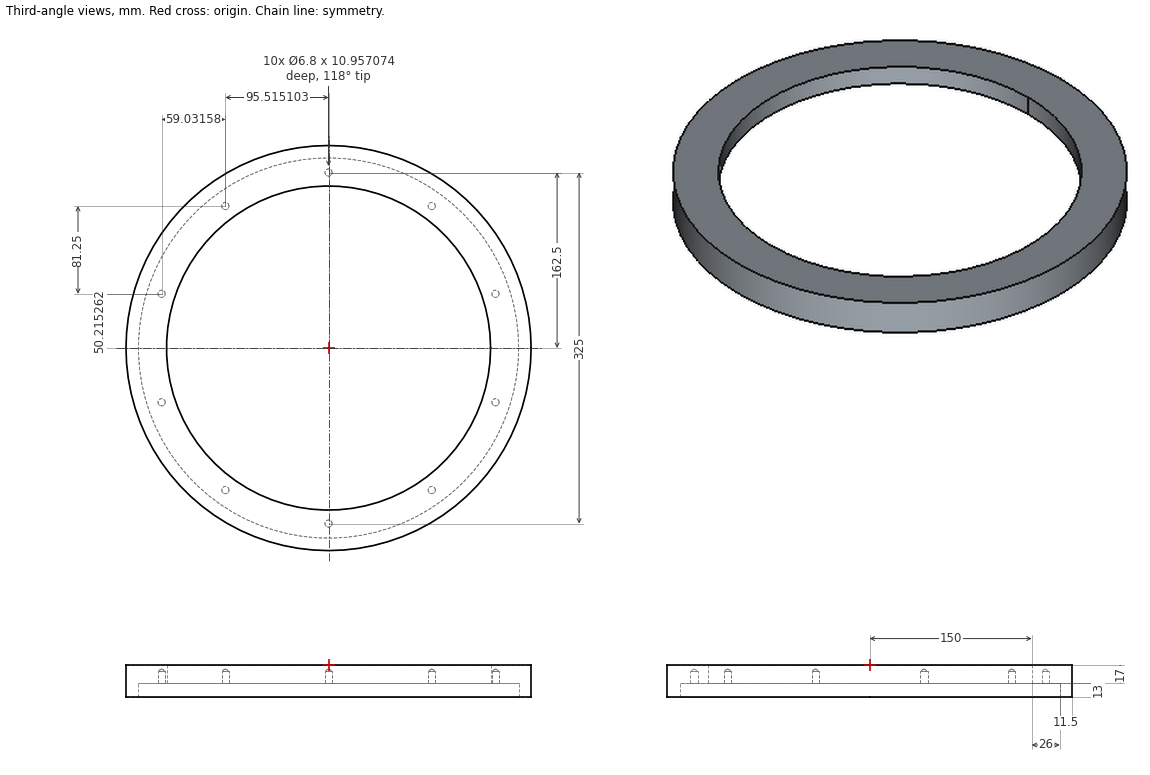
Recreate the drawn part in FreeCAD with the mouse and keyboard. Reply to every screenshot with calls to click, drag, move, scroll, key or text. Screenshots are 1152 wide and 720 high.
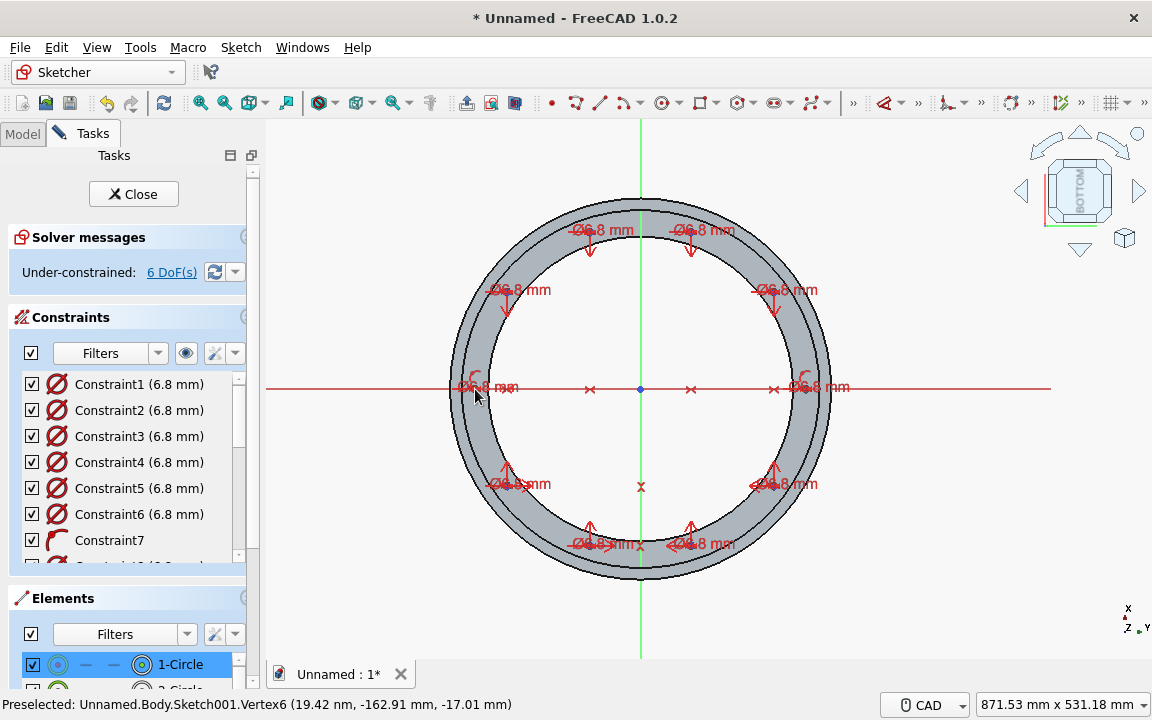
key(l)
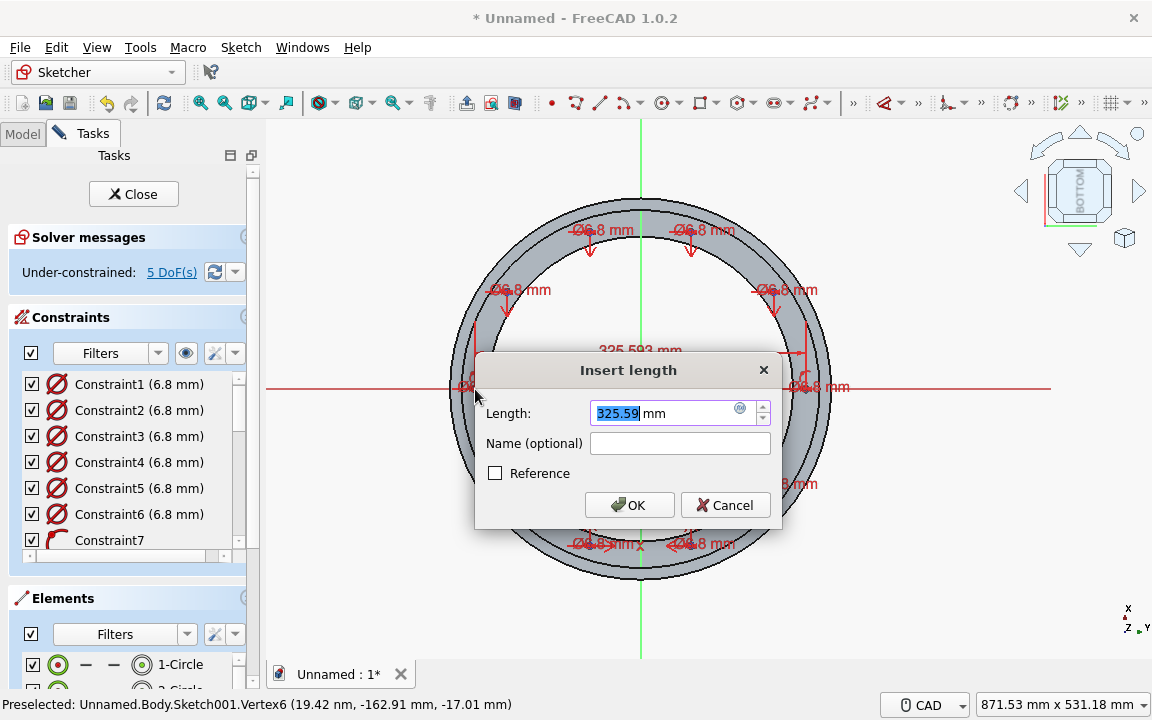
text(325)
key(Return)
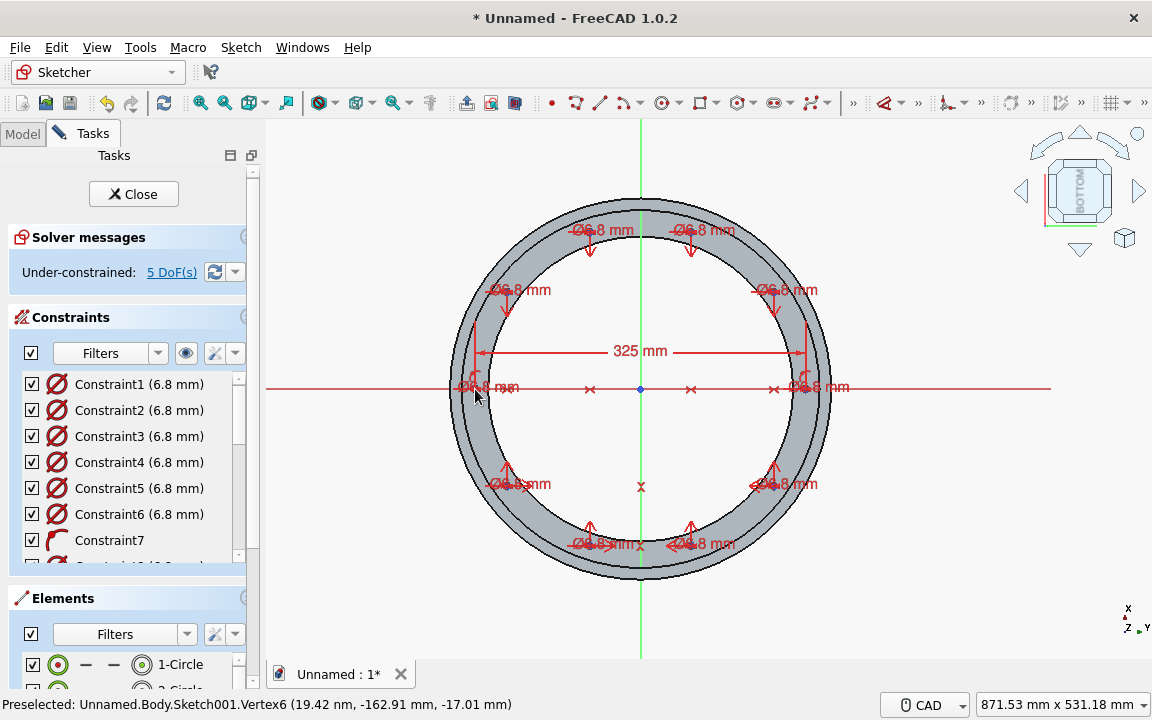
click(806, 389)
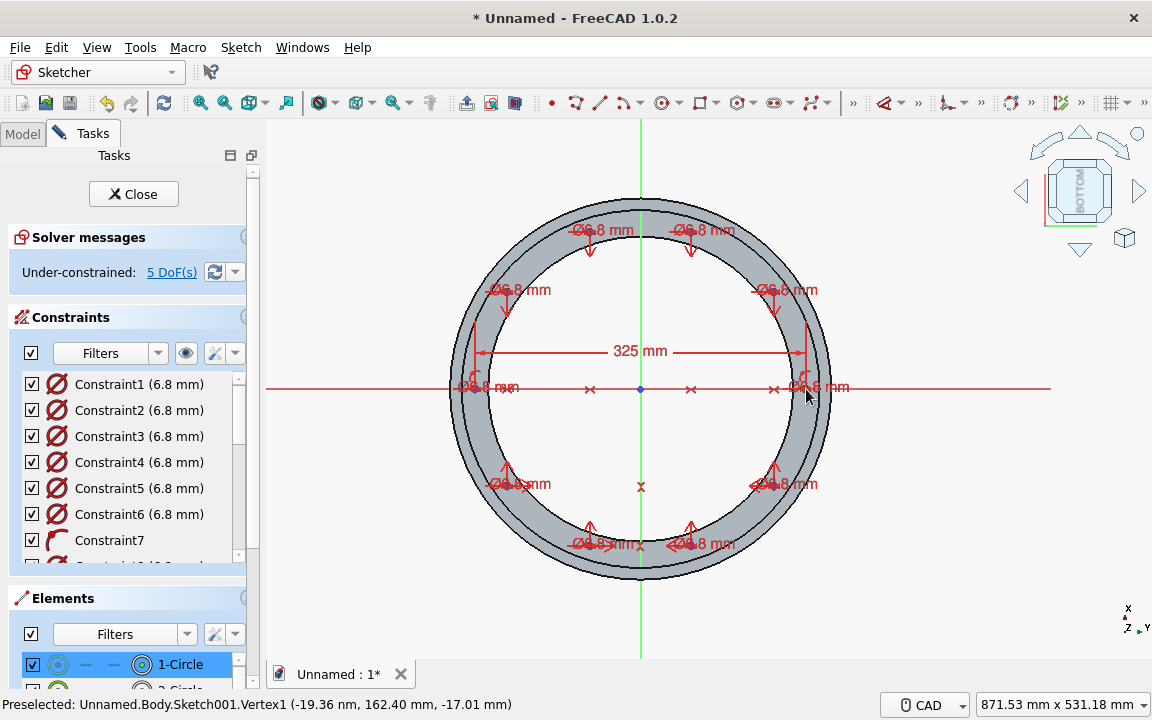
key(l)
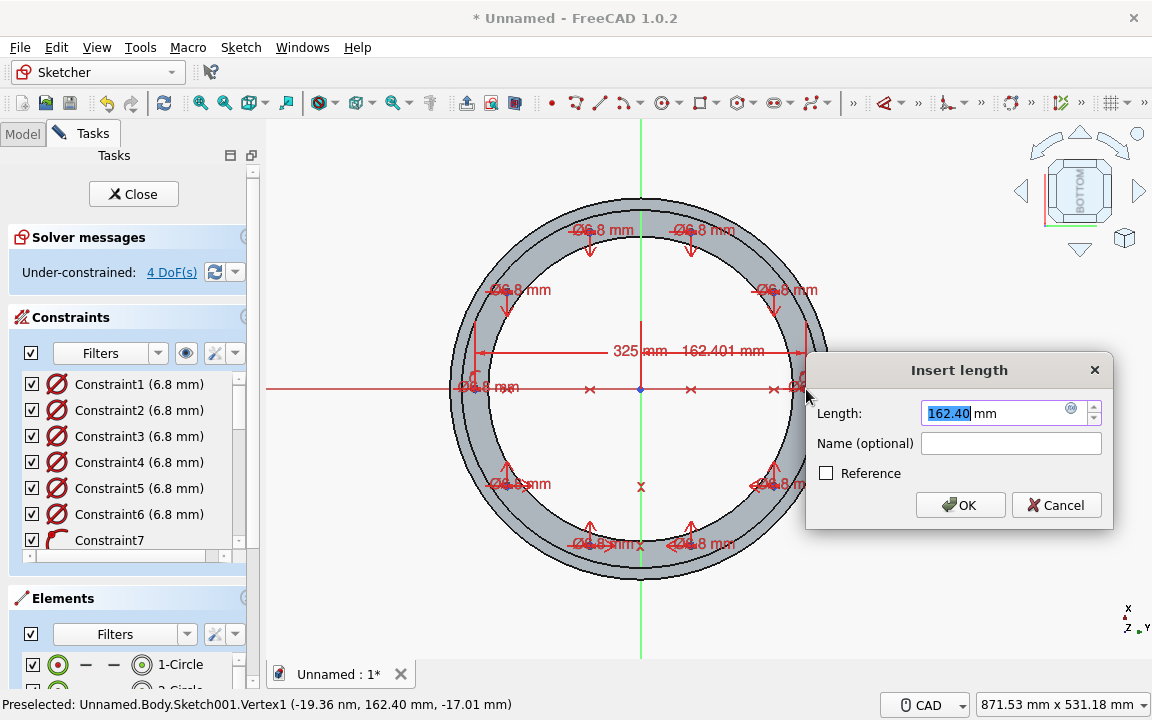
text(162.5)
key(Return)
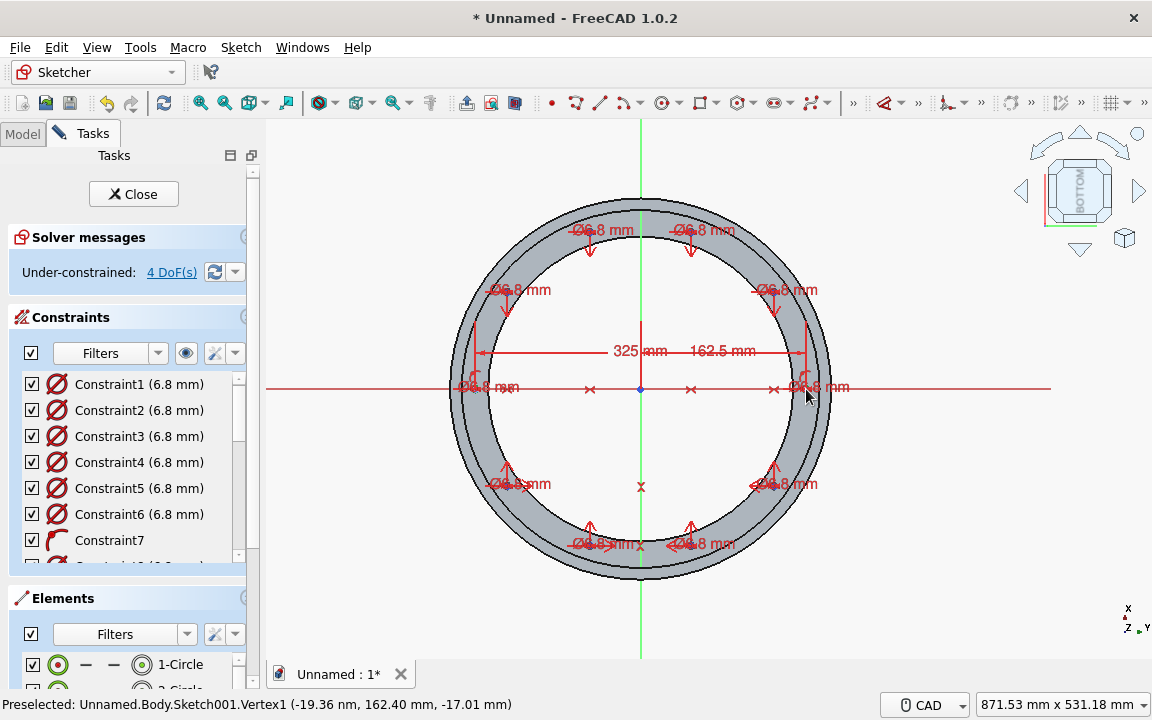
click(774, 486)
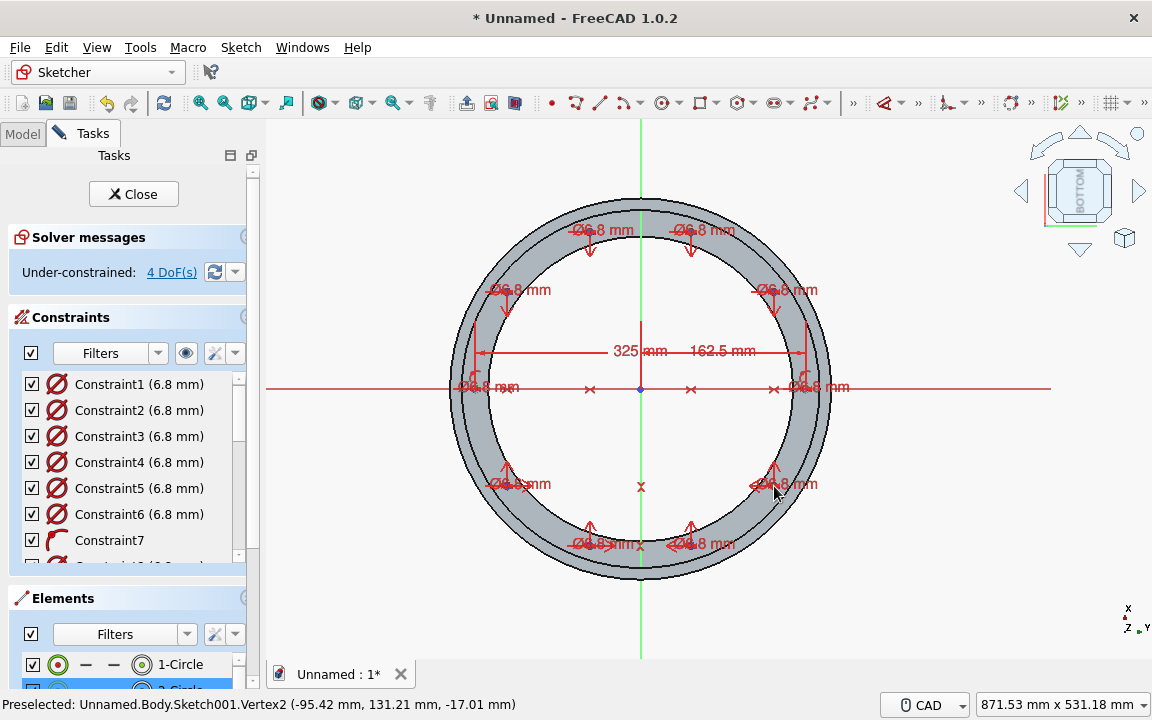
click(691, 546)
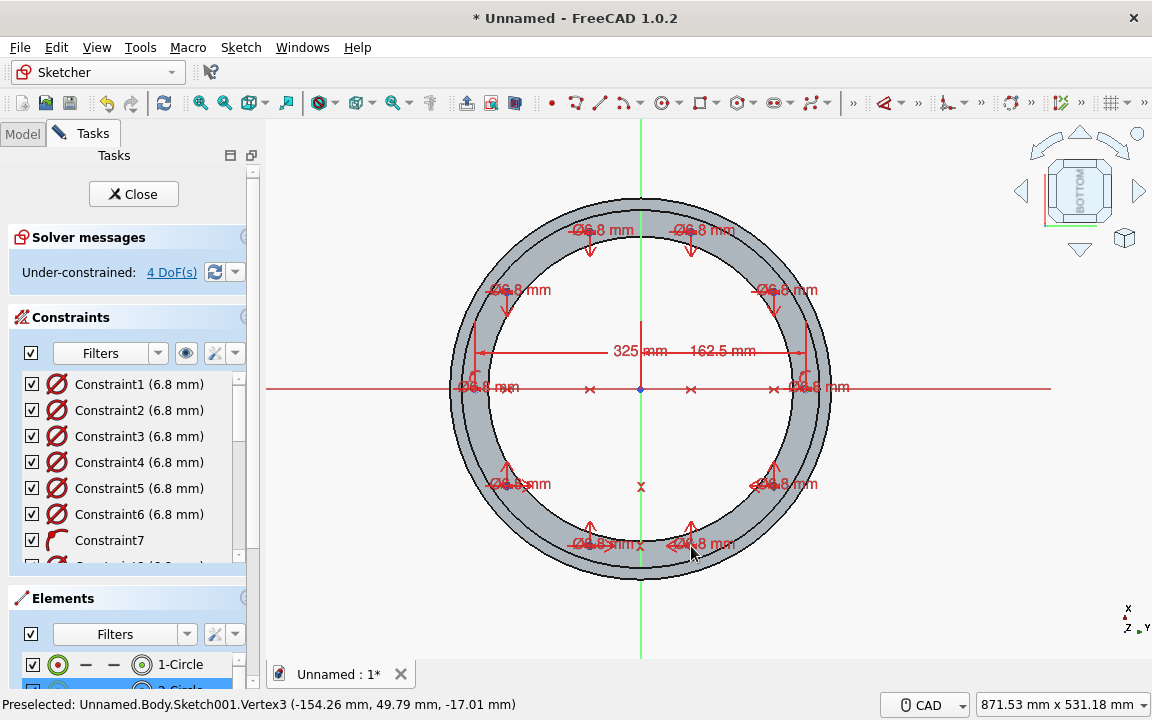
key(l)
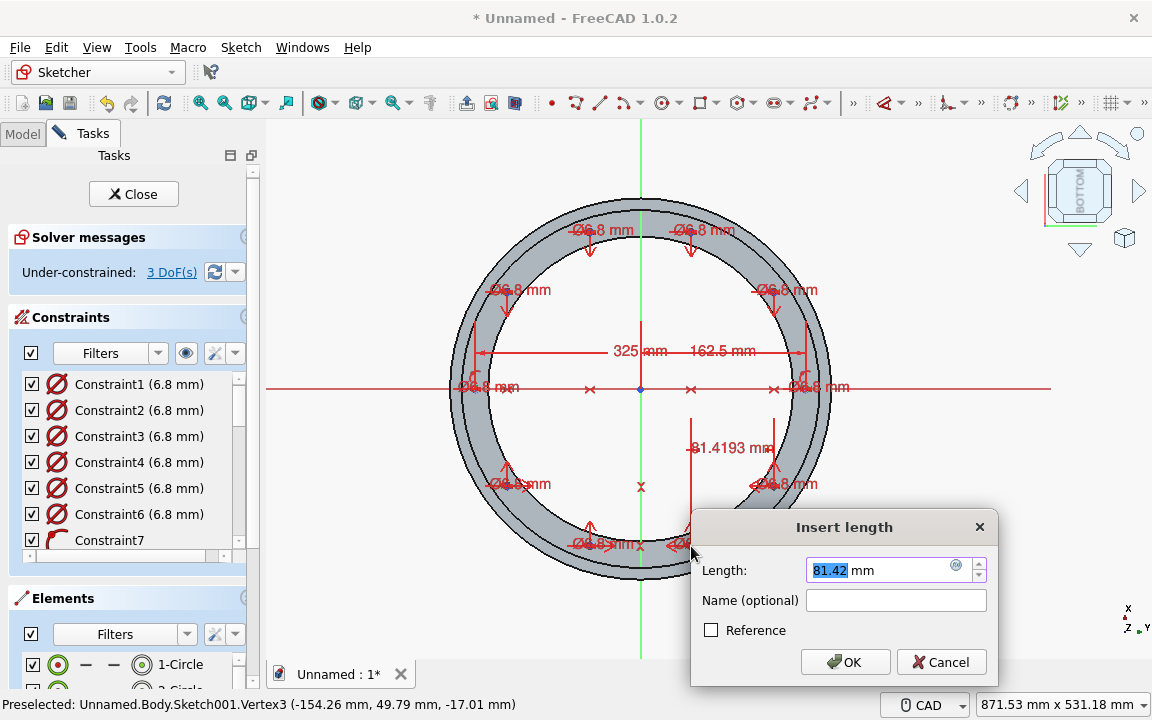
text(81.25)
key(Return)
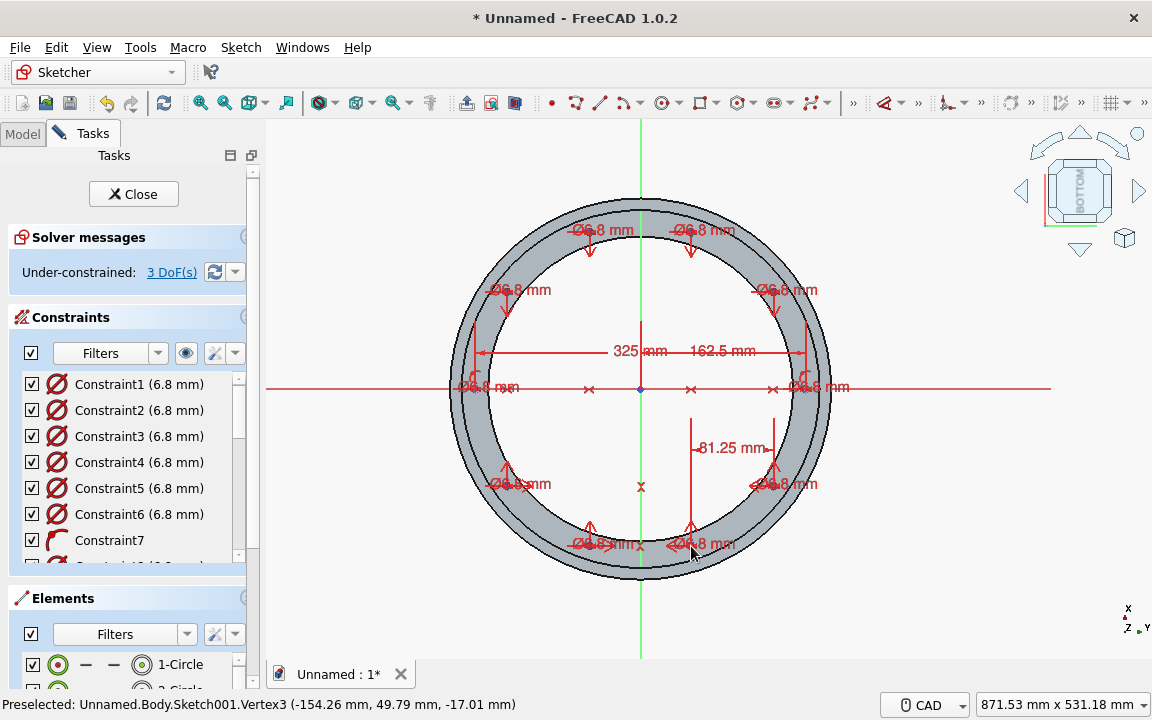
click(774, 486)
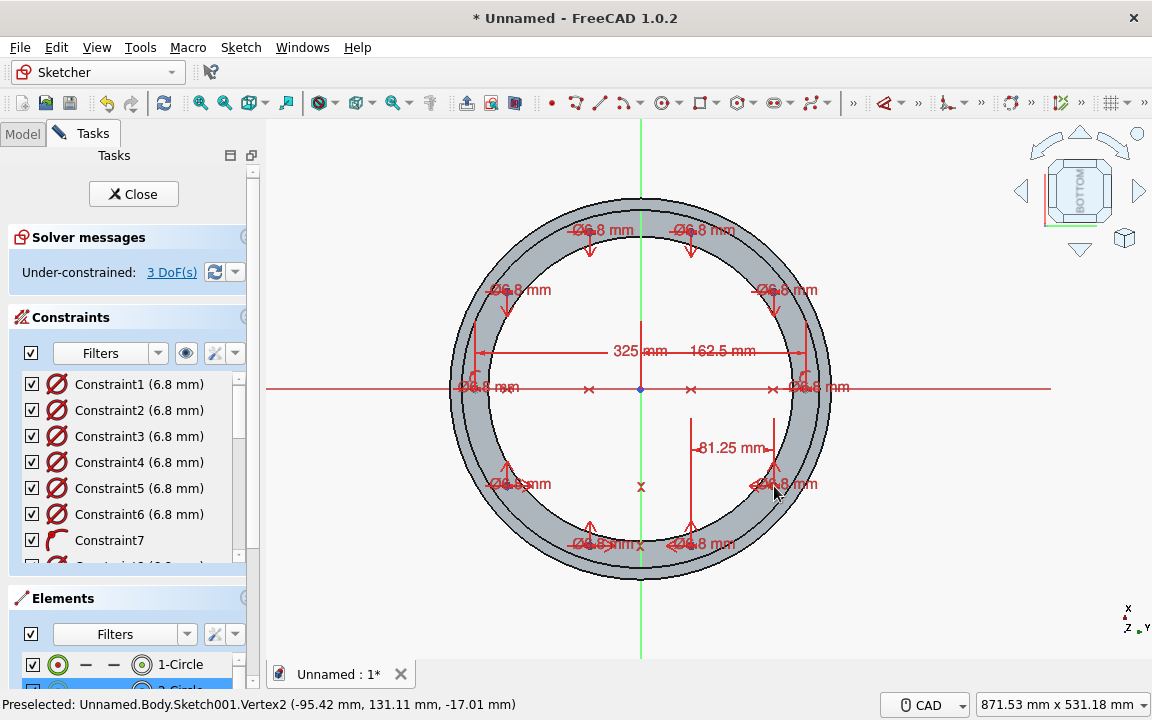
key(i)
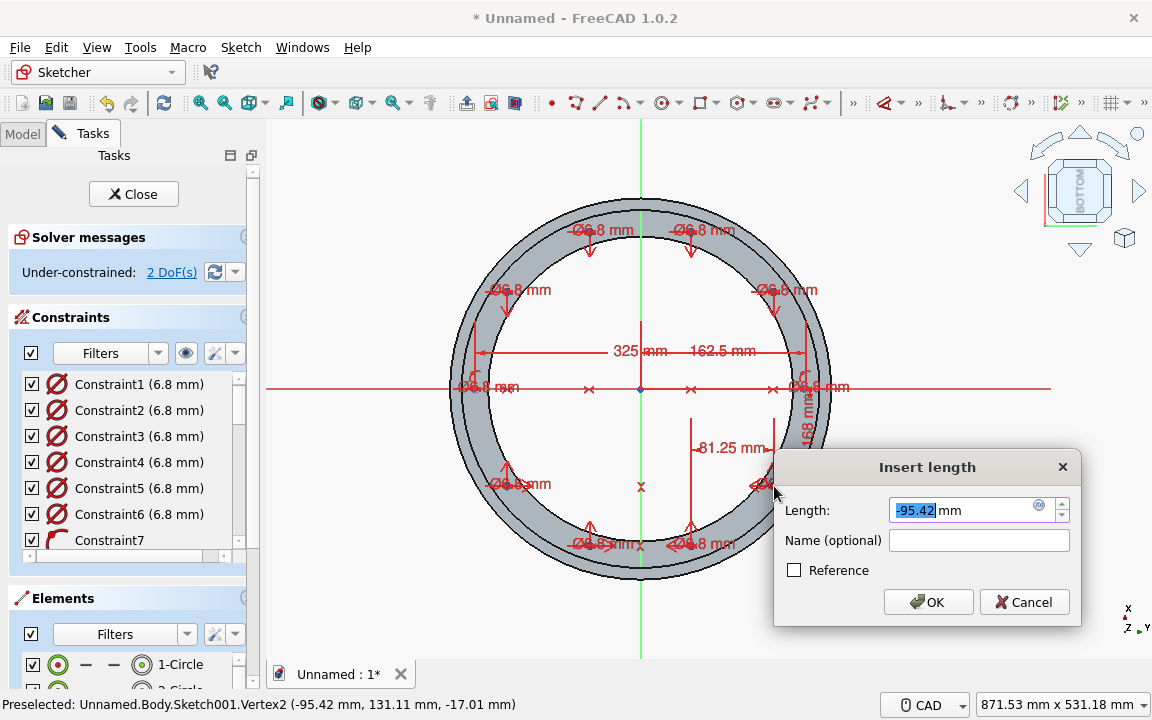
text(-95.515103)
key(Return)